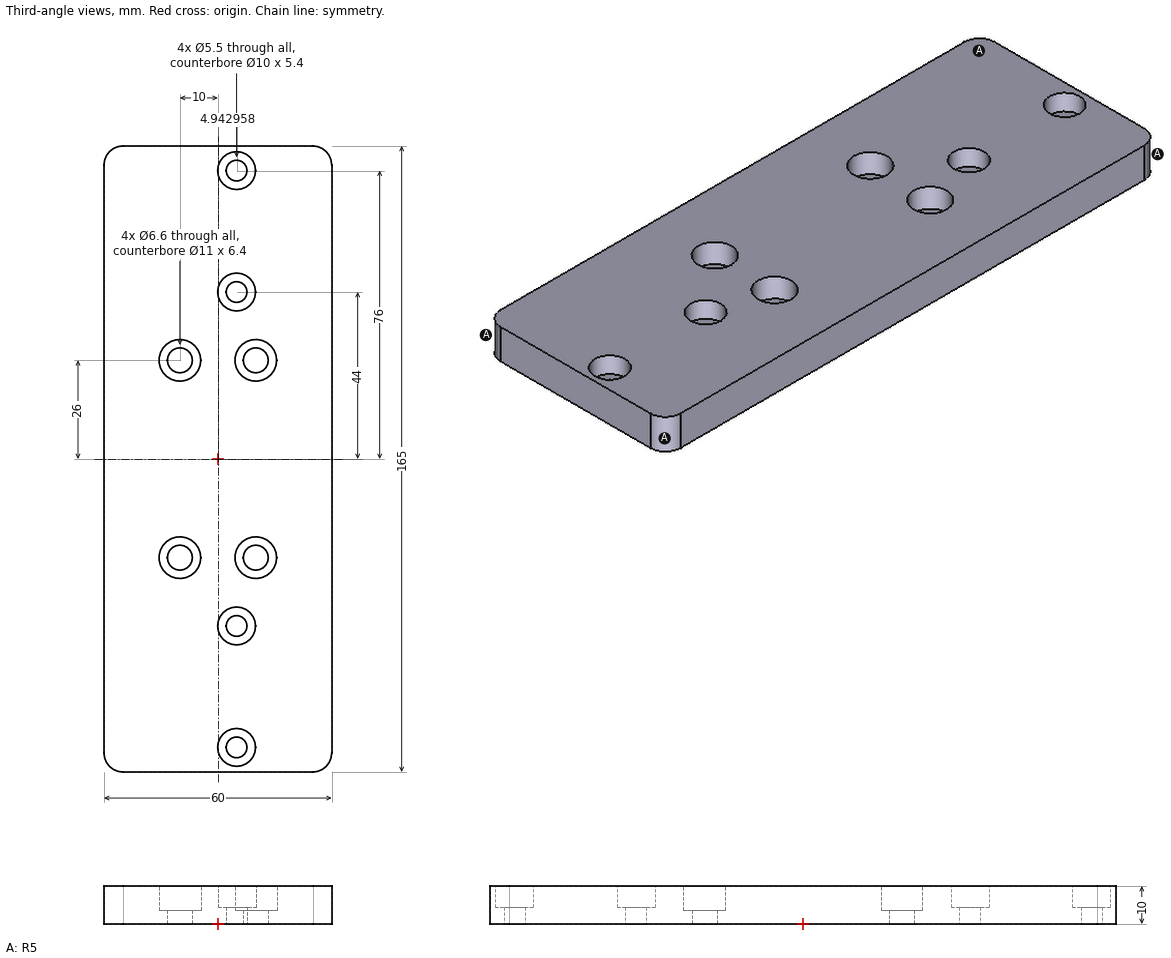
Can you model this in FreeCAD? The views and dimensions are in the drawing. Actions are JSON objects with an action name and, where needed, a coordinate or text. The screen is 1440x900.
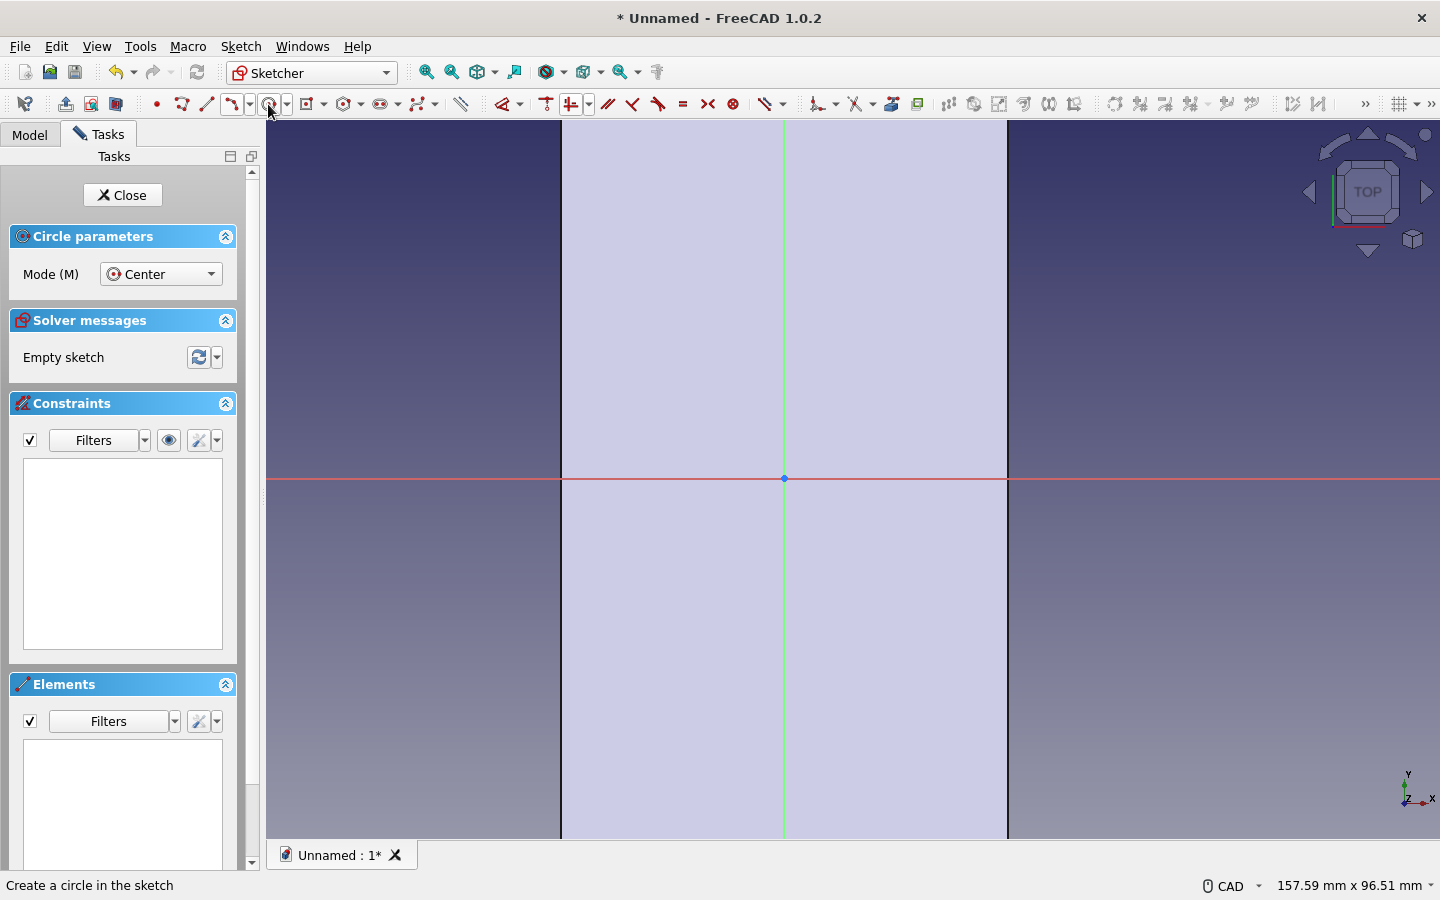
{"action": "left_click", "coordinate": [710, 285]}
{"action": "left_click", "coordinate": [727, 268]}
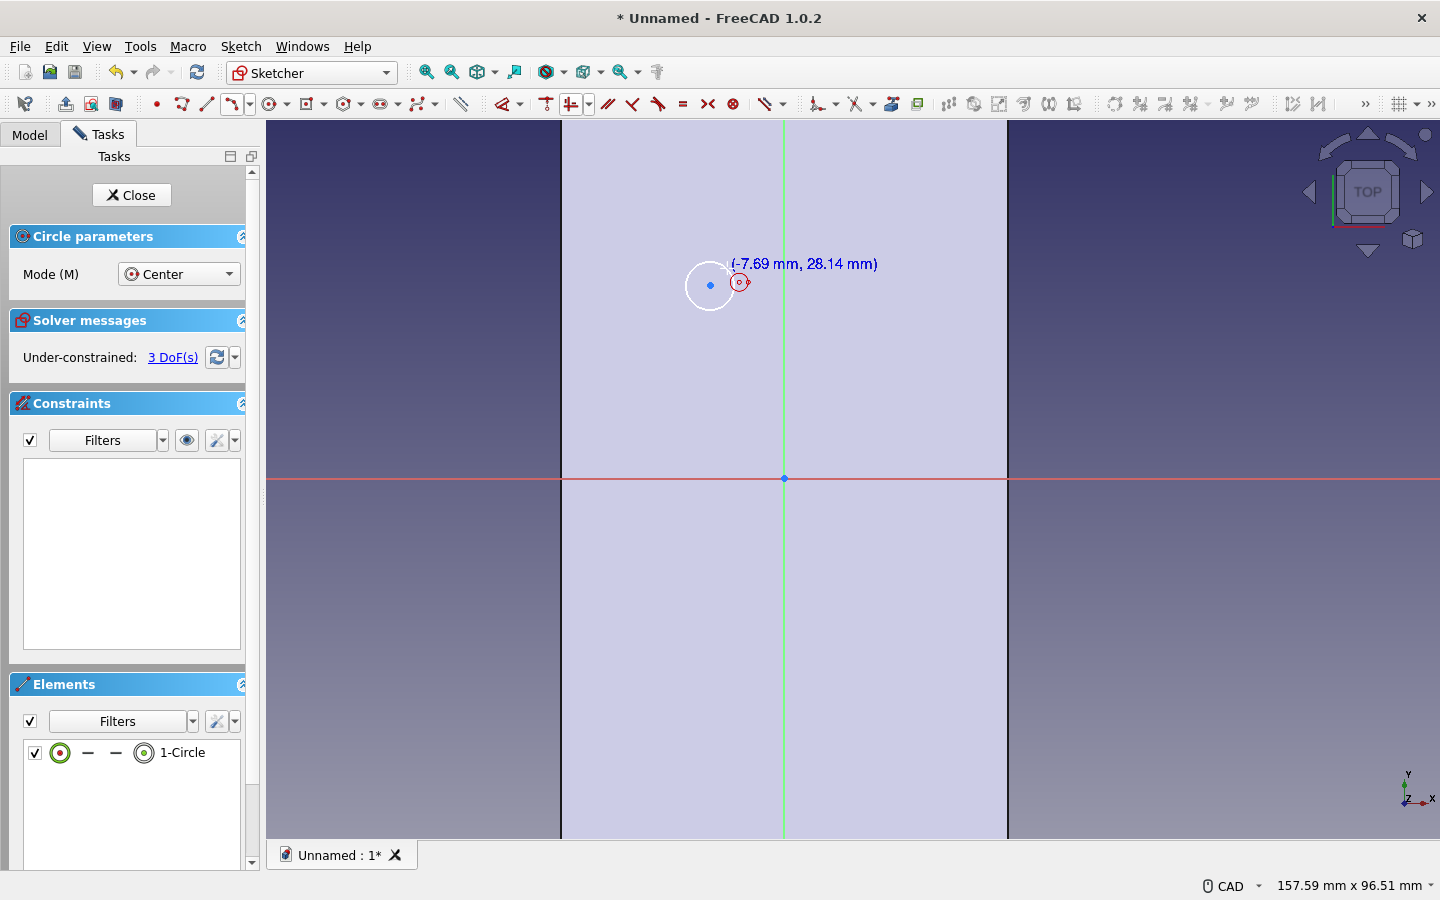
{"action": "left_click", "coordinate": [859, 285]}
{"action": "left_click", "coordinate": [876, 268]}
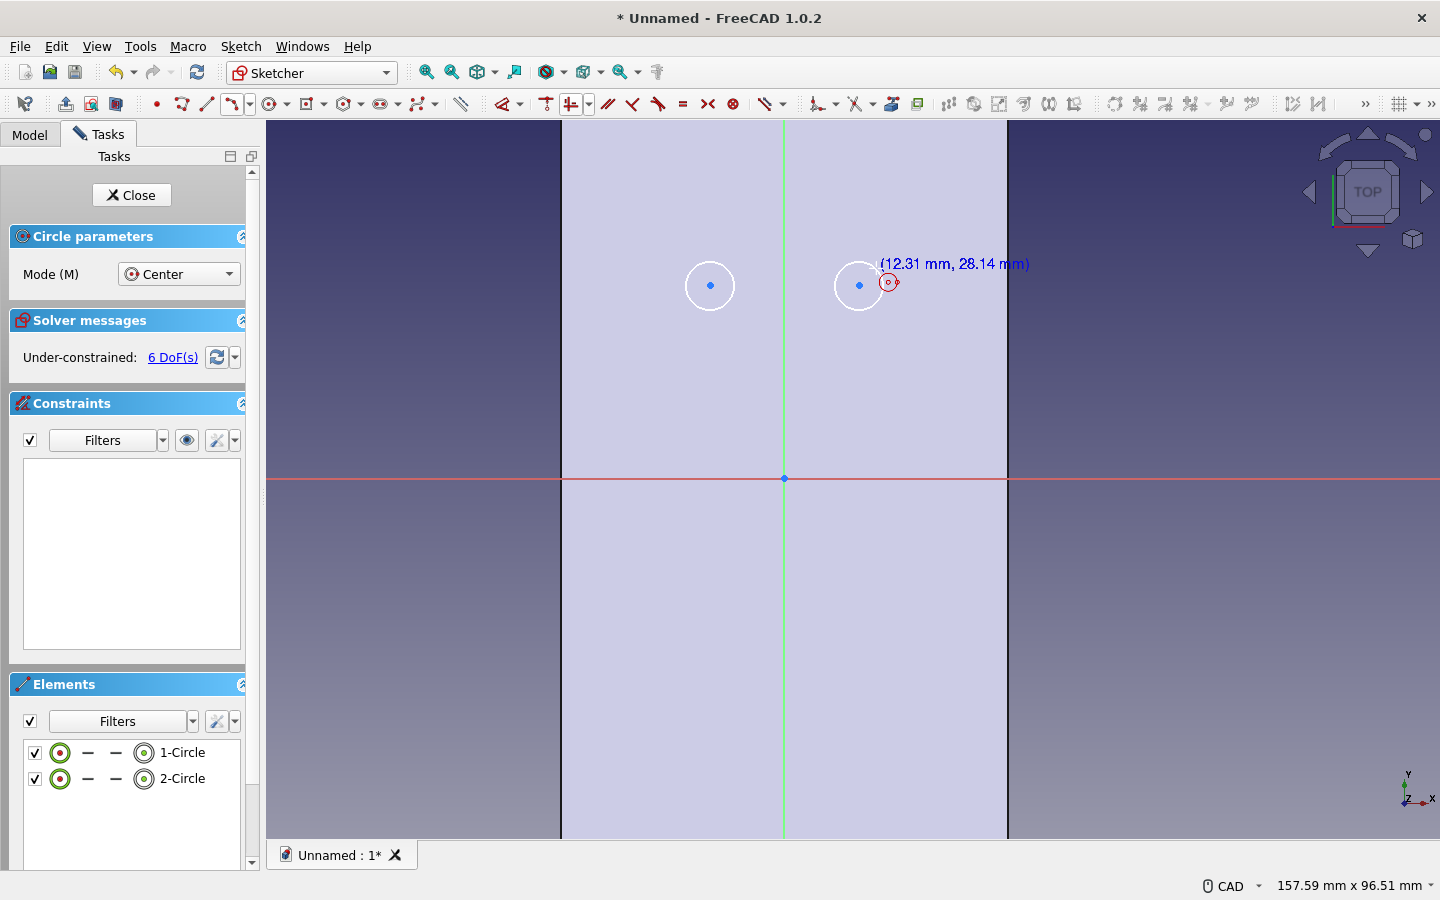
{"action": "left_click", "coordinate": [859, 672]}
{"action": "left_click", "coordinate": [876, 655]}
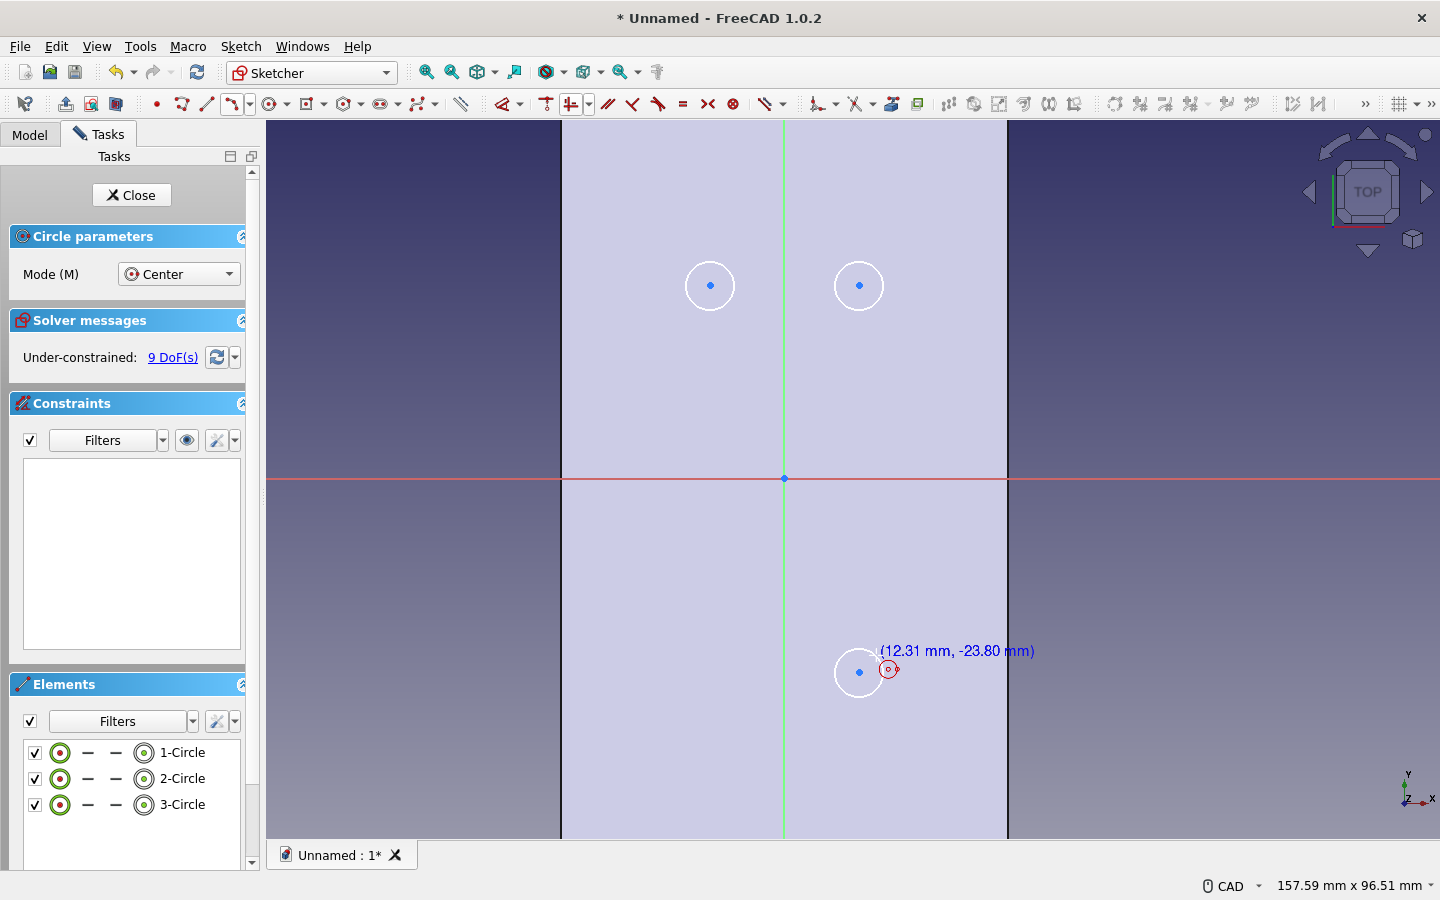
{"action": "left_click", "coordinate": [710, 672]}
{"action": "left_click", "coordinate": [727, 655]}
{"action": "key", "text": "Escape"}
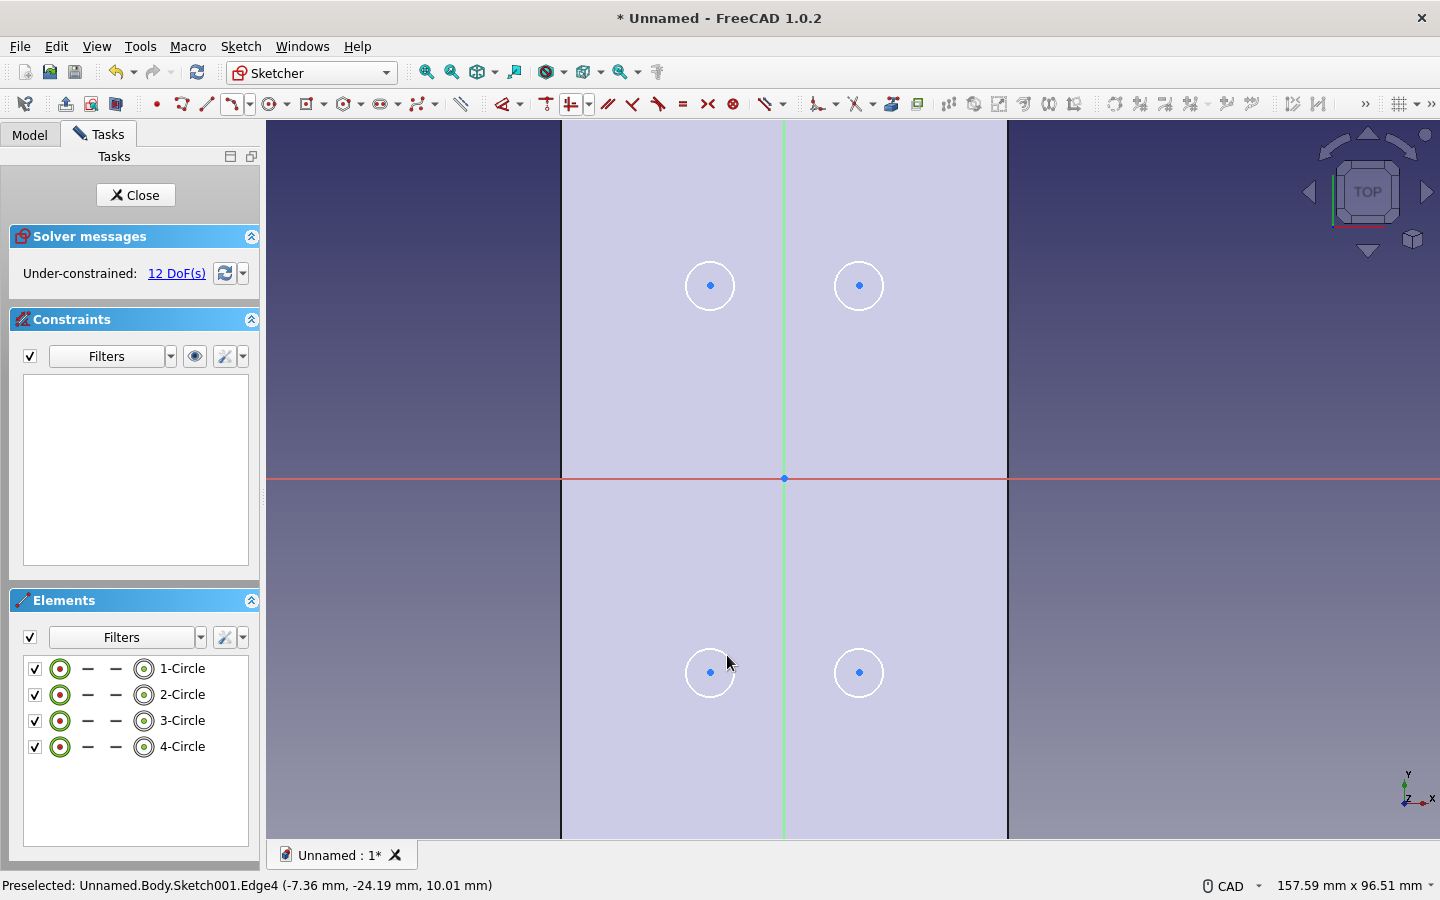
{"action": "left_click", "coordinate": [727, 269]}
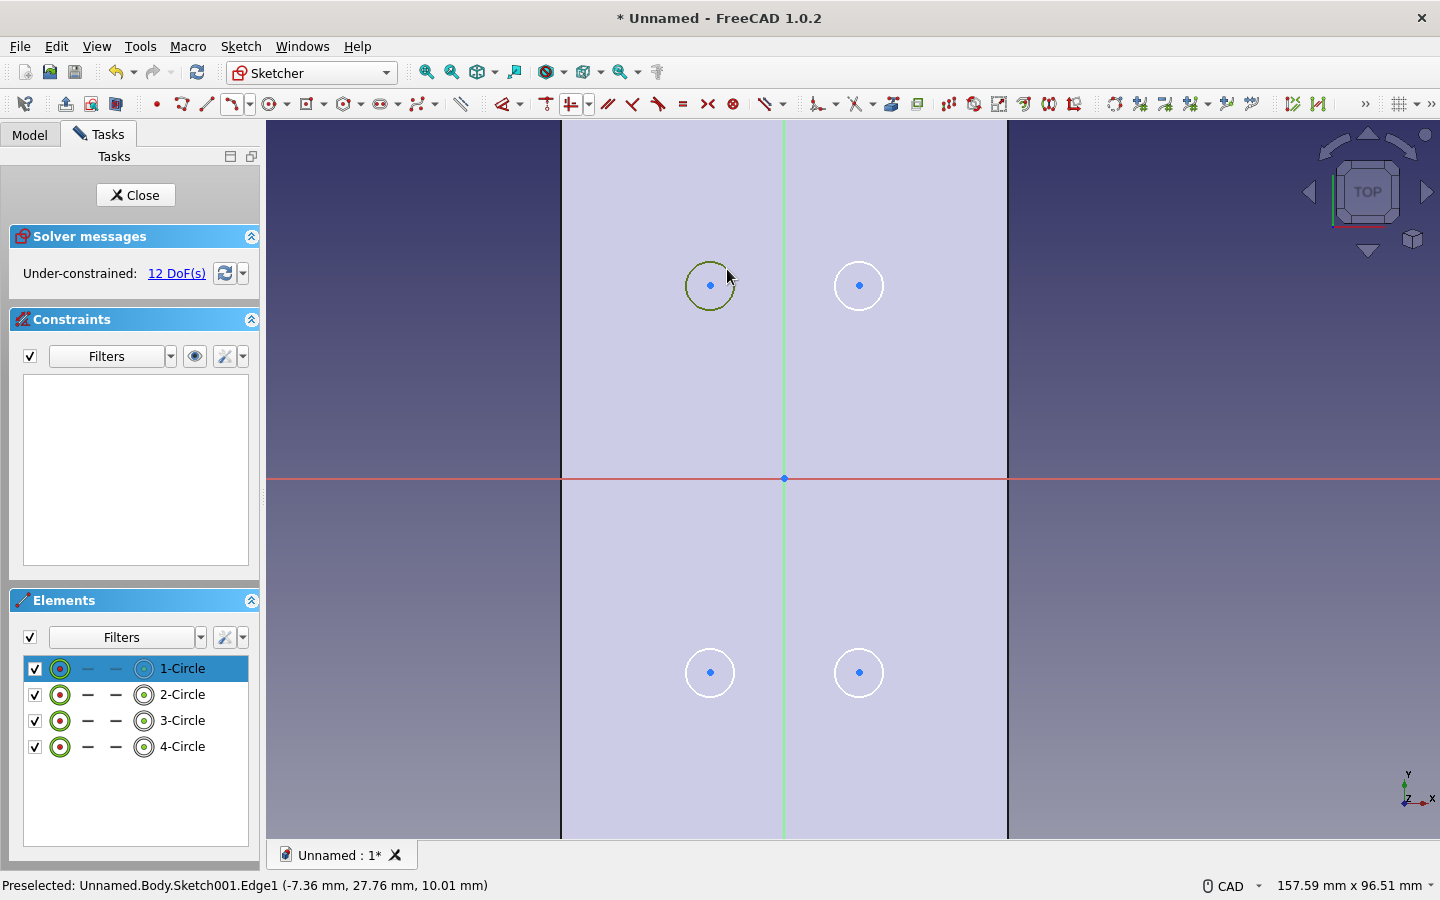
{"action": "left_click", "coordinate": [876, 269]}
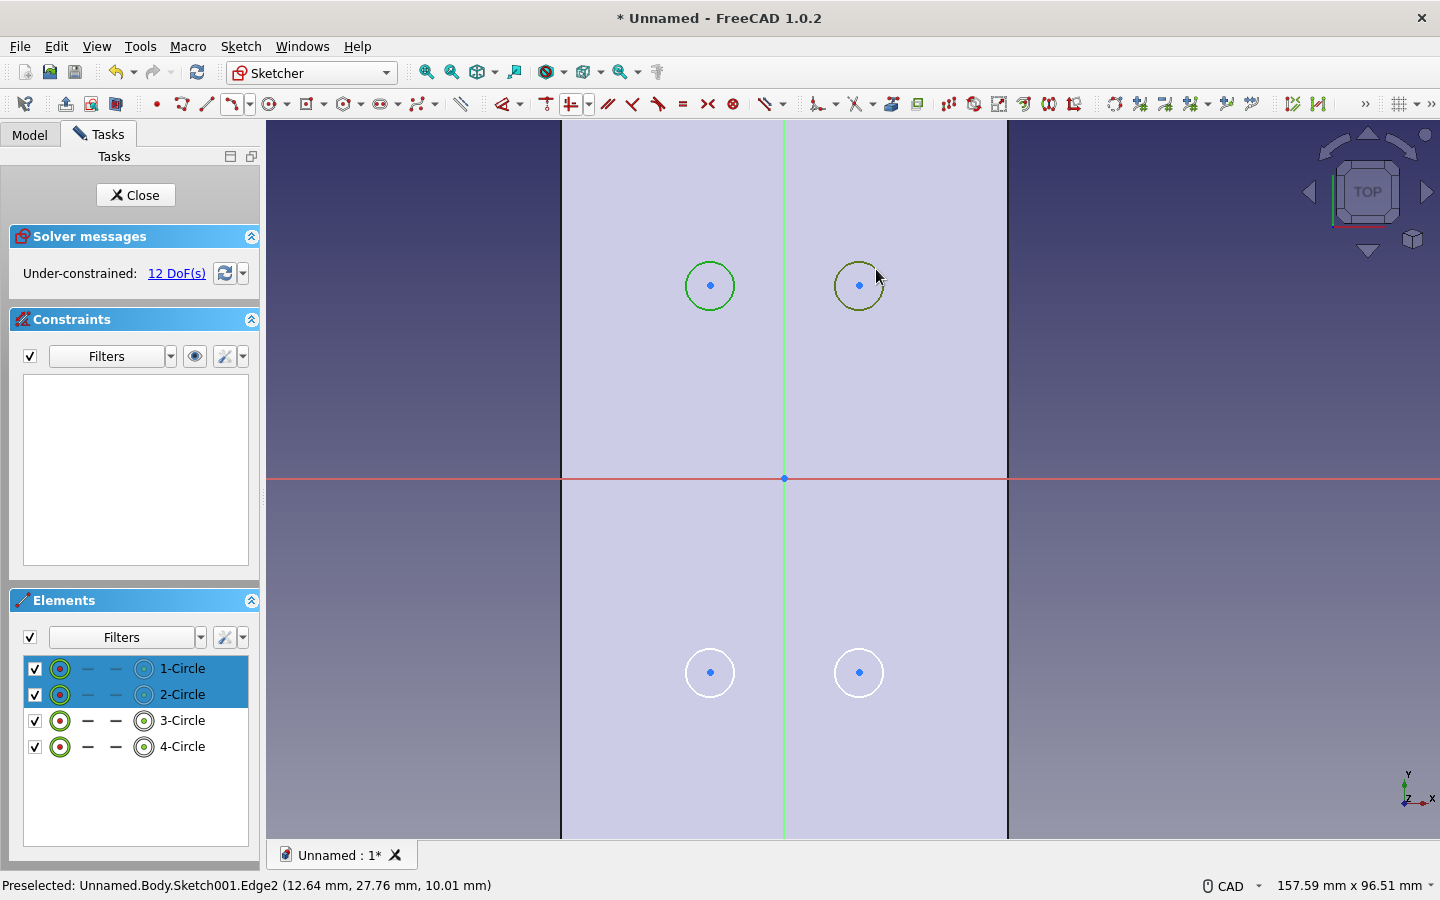
{"action": "left_click", "coordinate": [876, 656]}